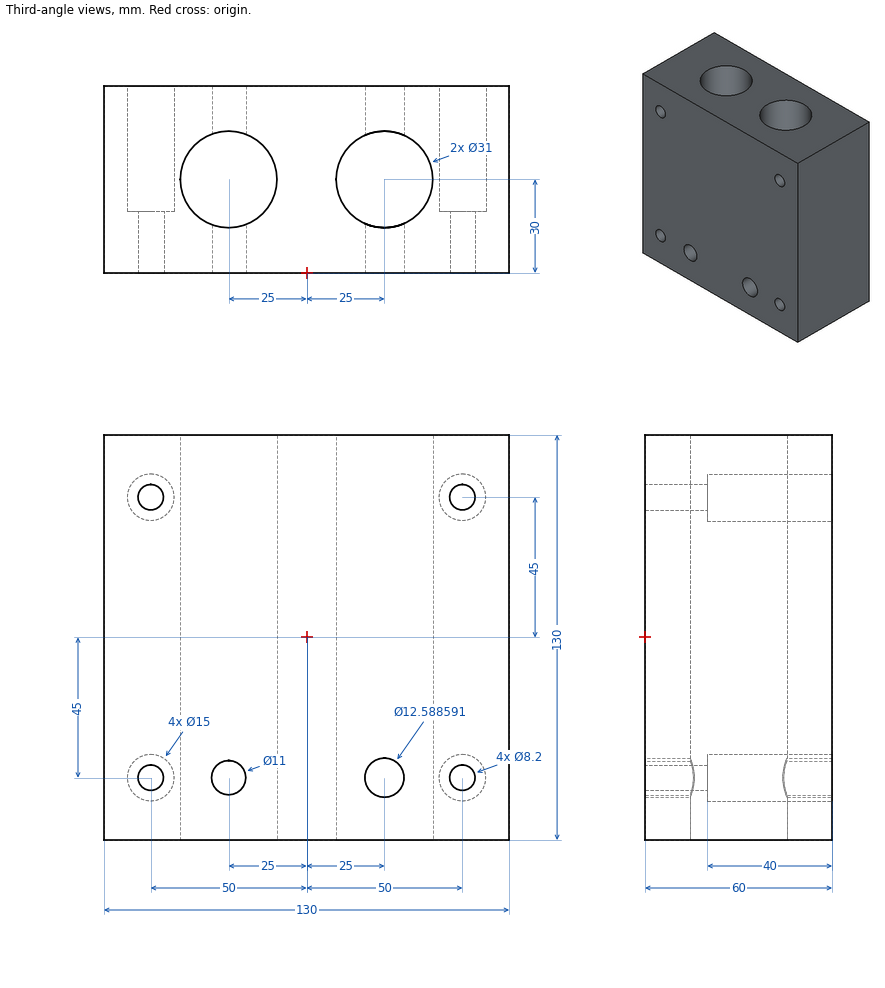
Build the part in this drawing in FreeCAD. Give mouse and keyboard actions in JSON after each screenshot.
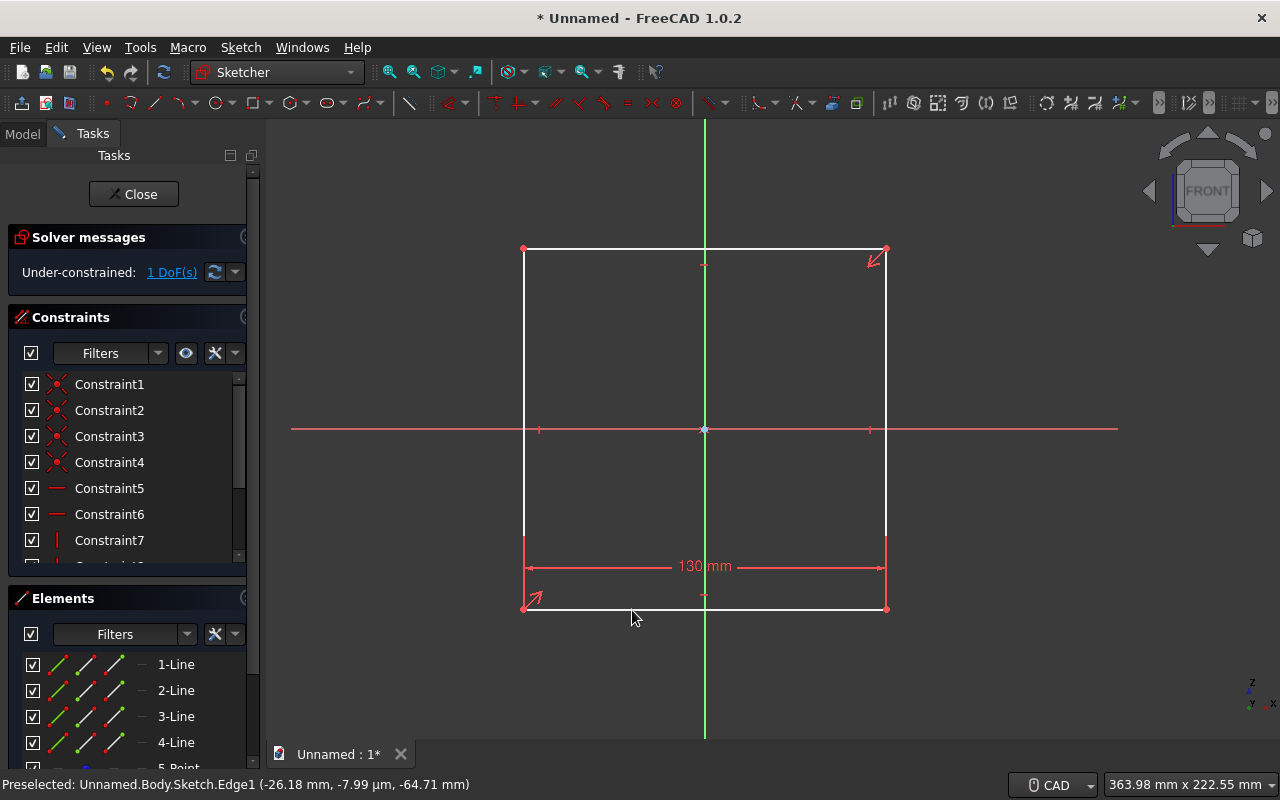
{"action": "left_click", "coordinate": [886, 501]}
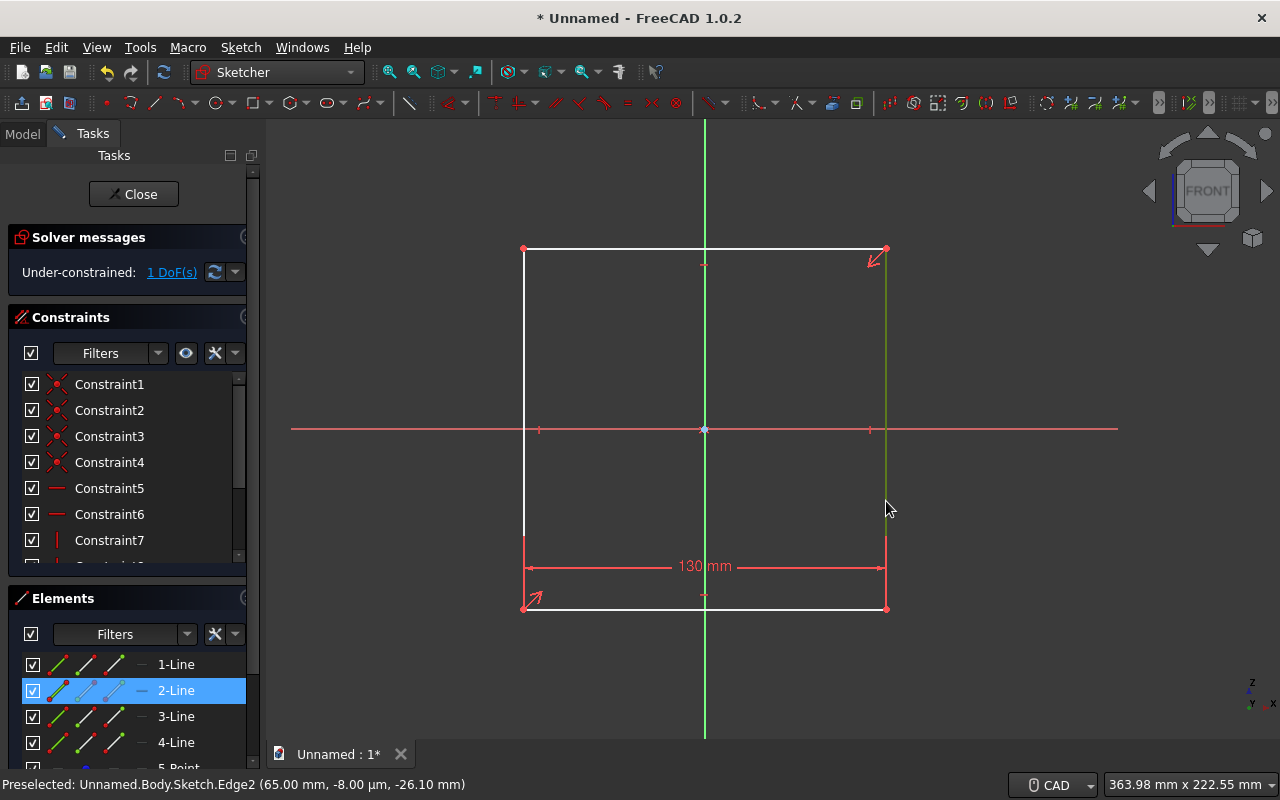
{"action": "key", "text": "i"}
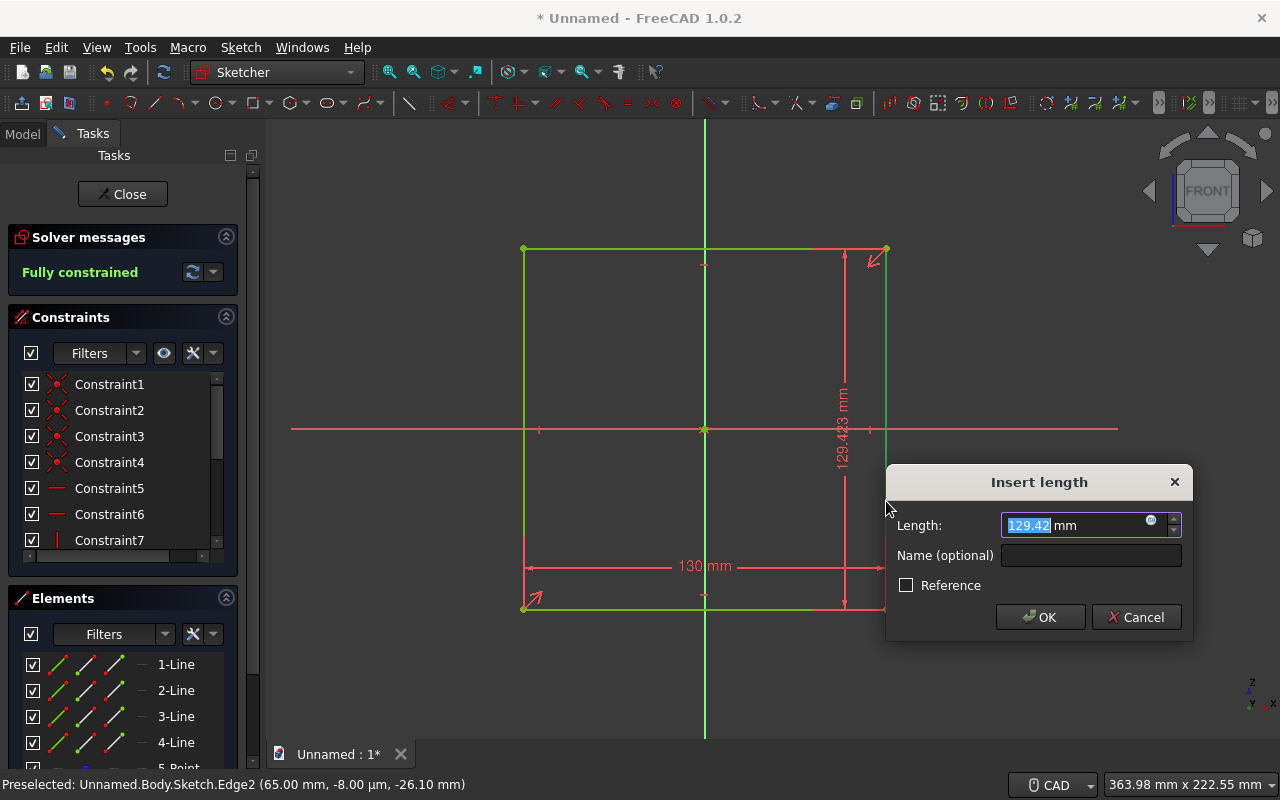
{"action": "type", "text": "130"}
{"action": "key", "text": "Return"}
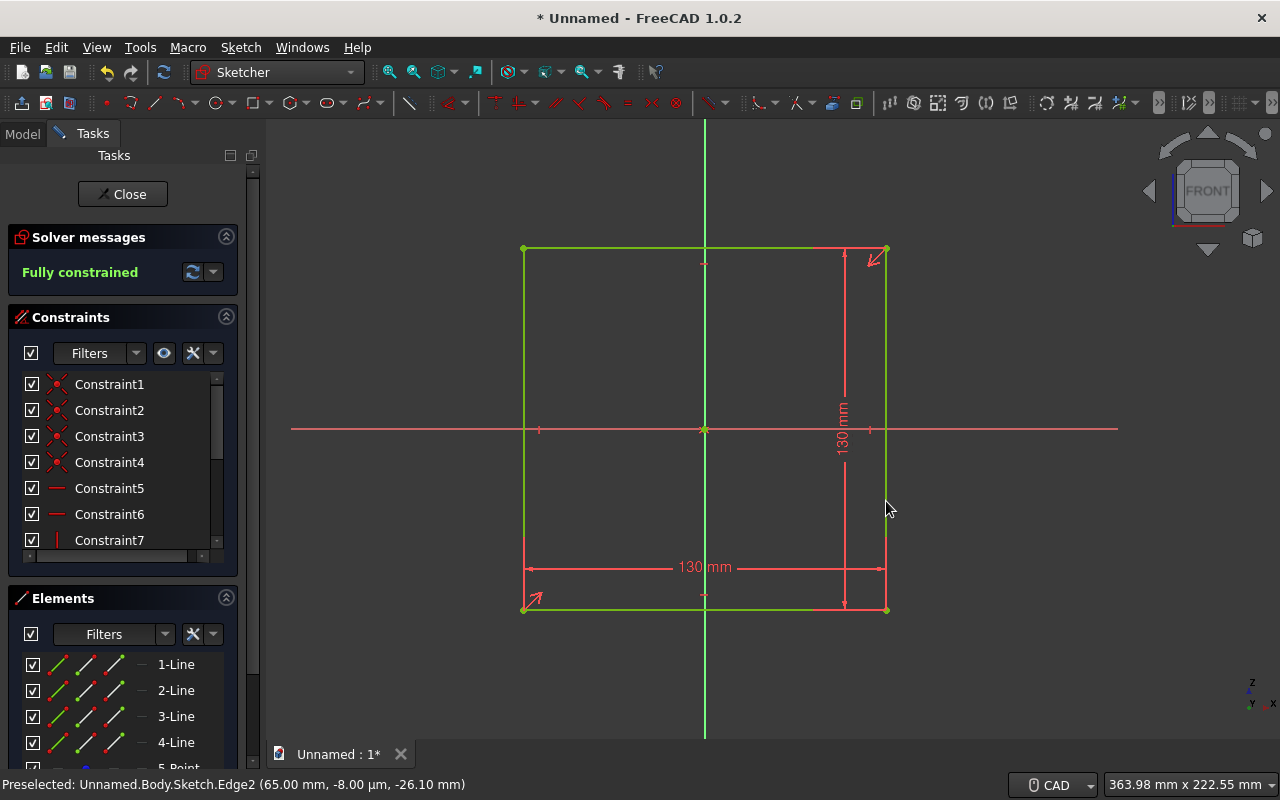
{"action": "left_click", "coordinate": [123, 194]}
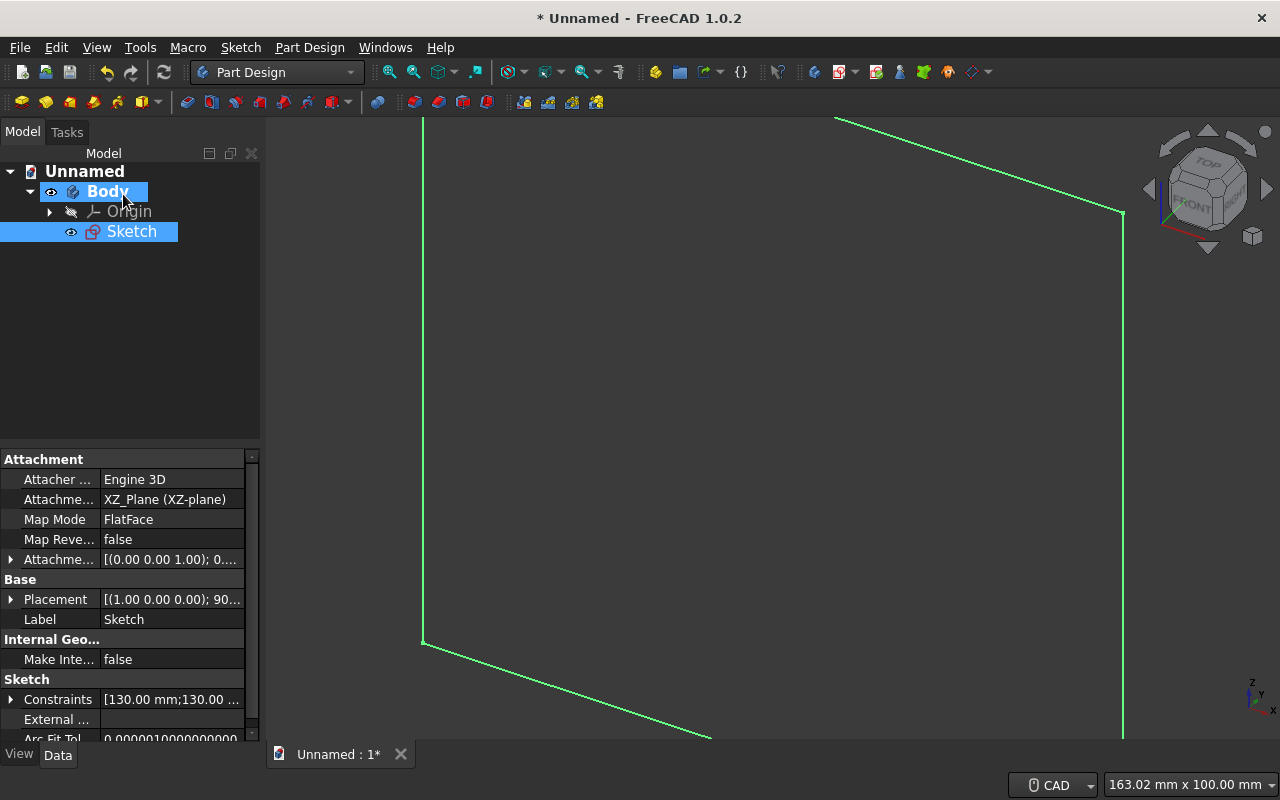
{"action": "left_click", "coordinate": [22, 102]}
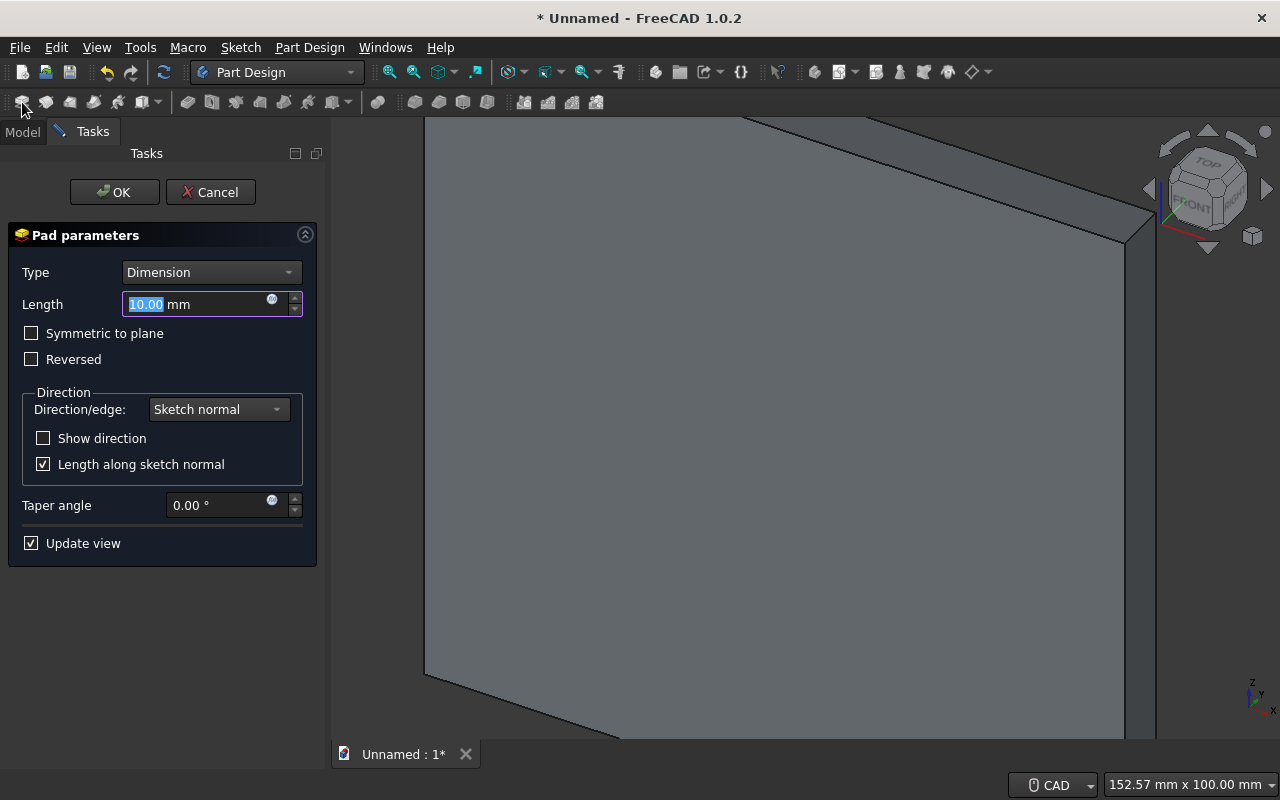
{"action": "type", "text": "60"}
{"action": "key", "text": "Tab"}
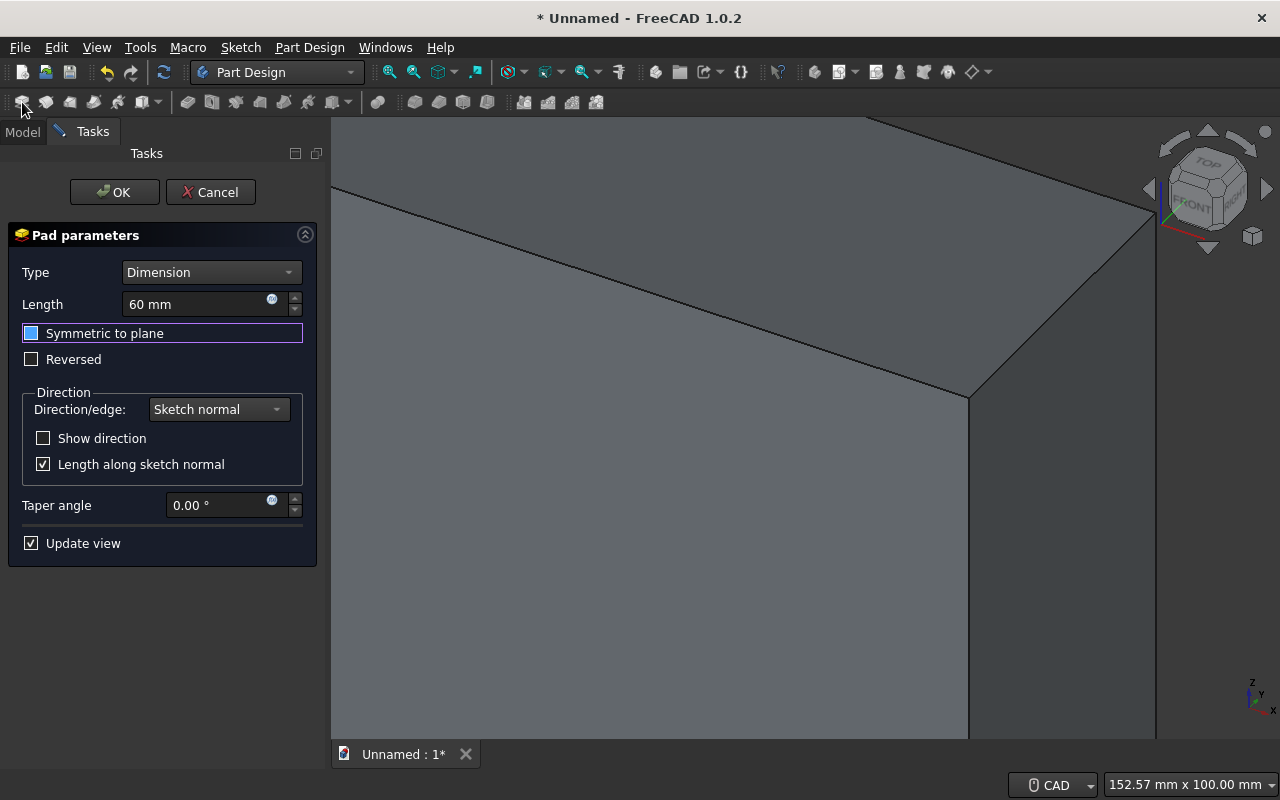
{"action": "left_click", "coordinate": [30, 359]}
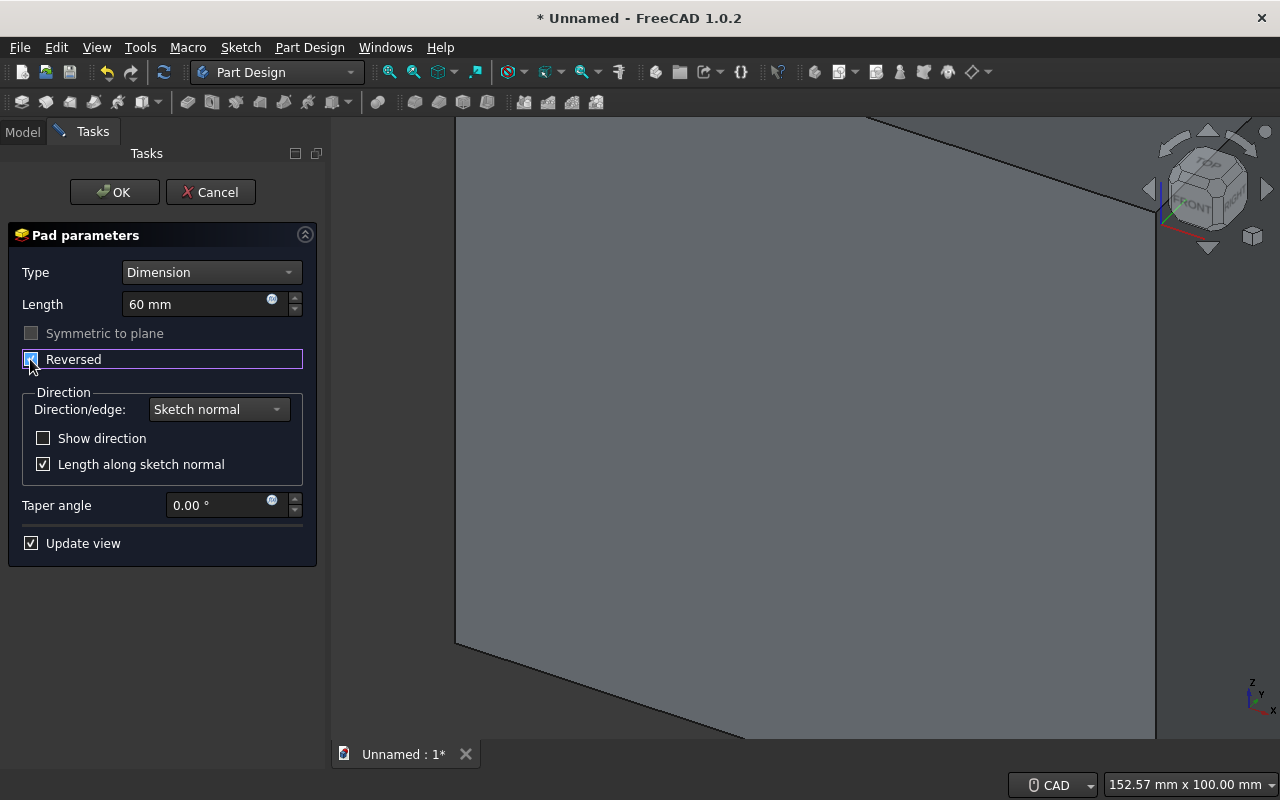
{"action": "left_click", "coordinate": [115, 192]}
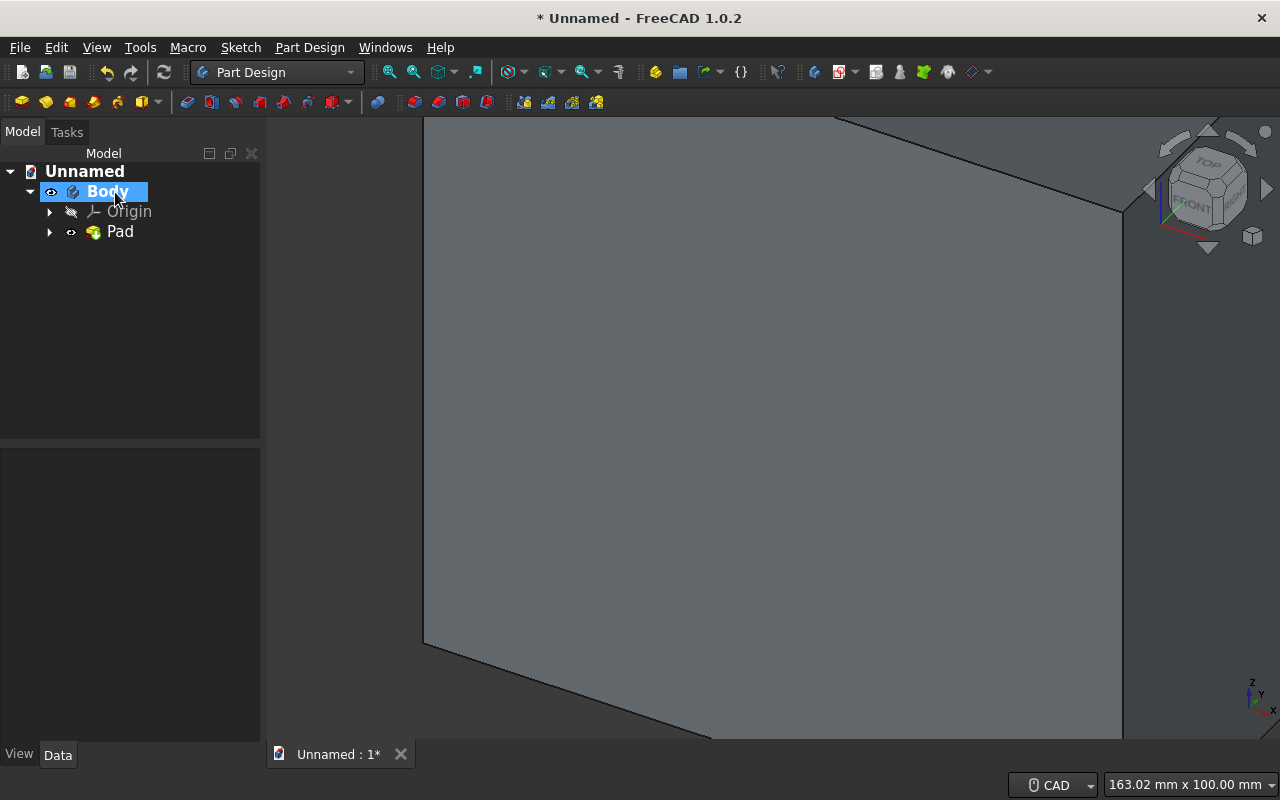
{"action": "left_click", "coordinate": [390, 72]}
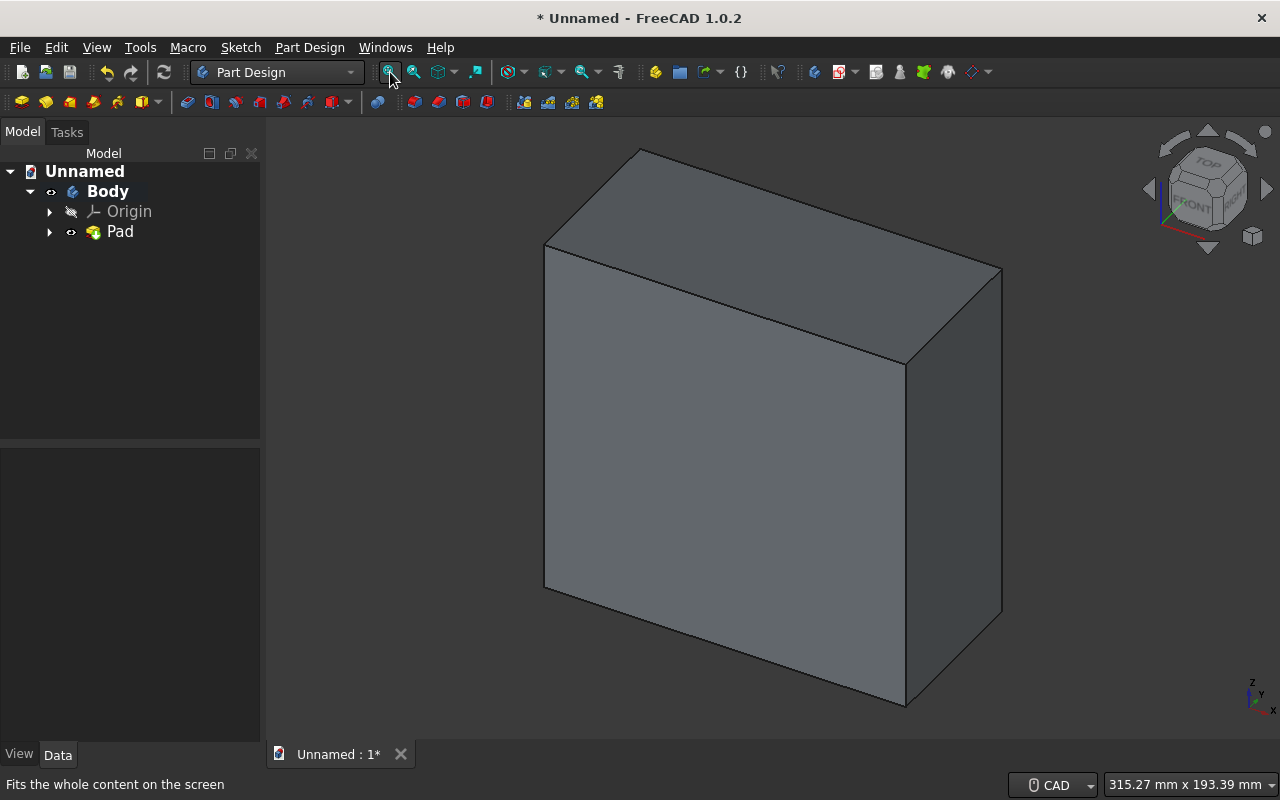
{"action": "key", "text": "5"}